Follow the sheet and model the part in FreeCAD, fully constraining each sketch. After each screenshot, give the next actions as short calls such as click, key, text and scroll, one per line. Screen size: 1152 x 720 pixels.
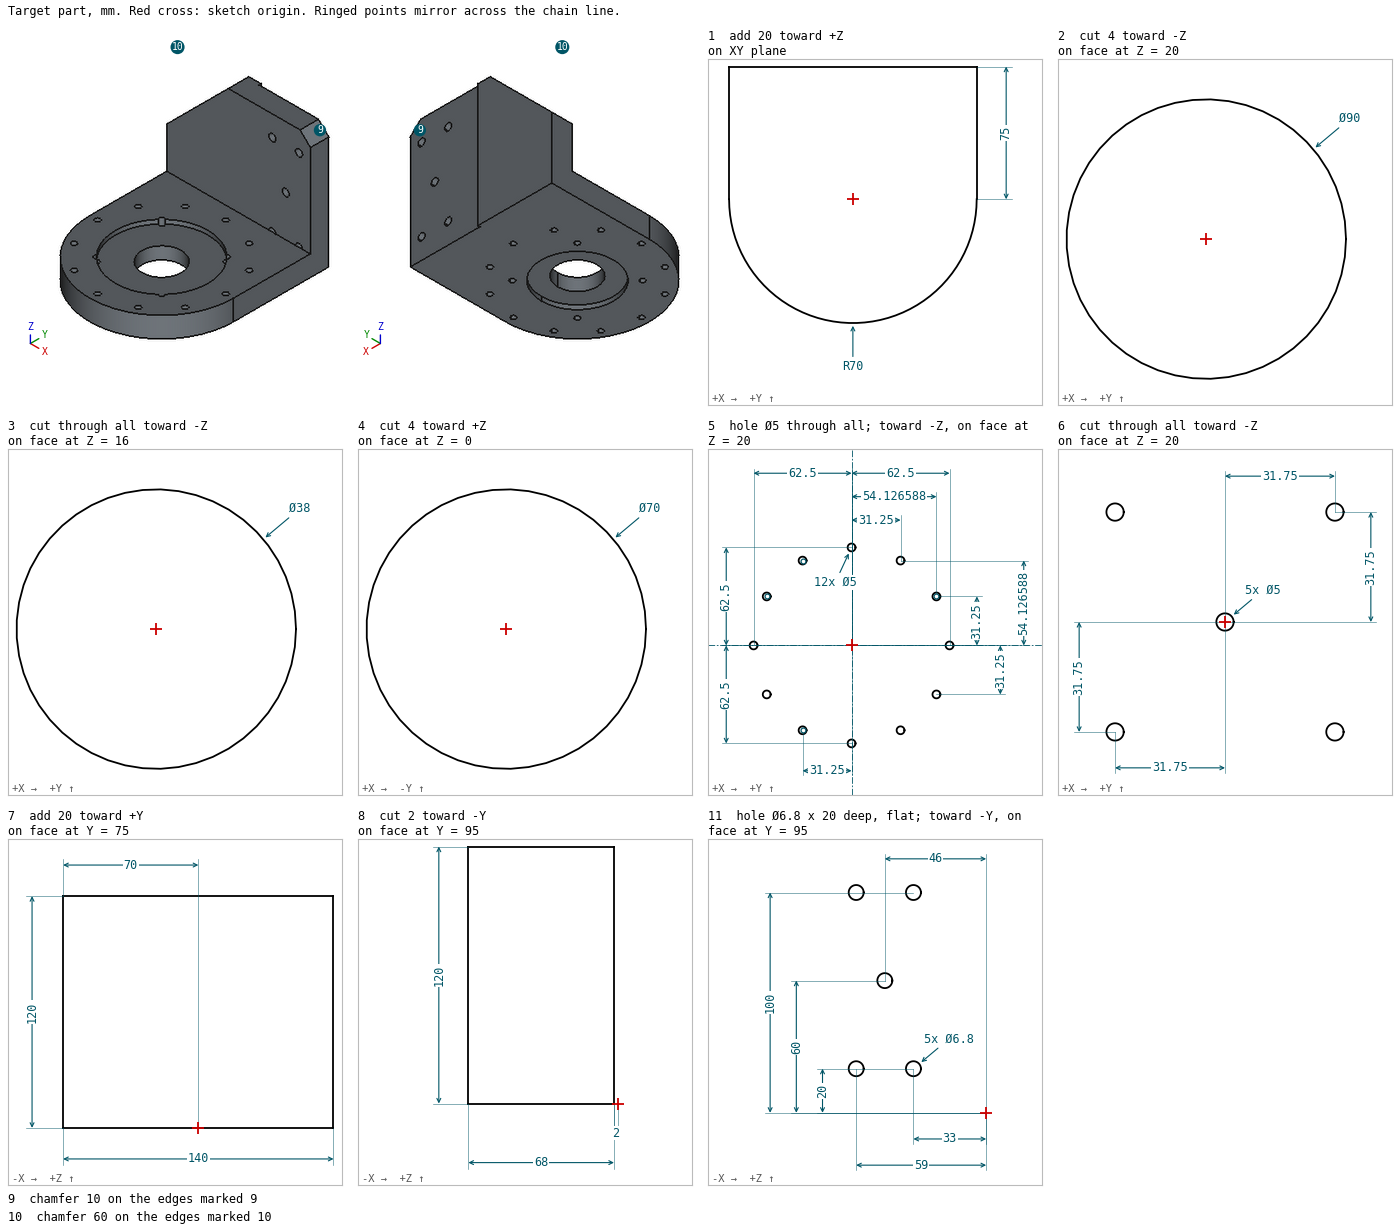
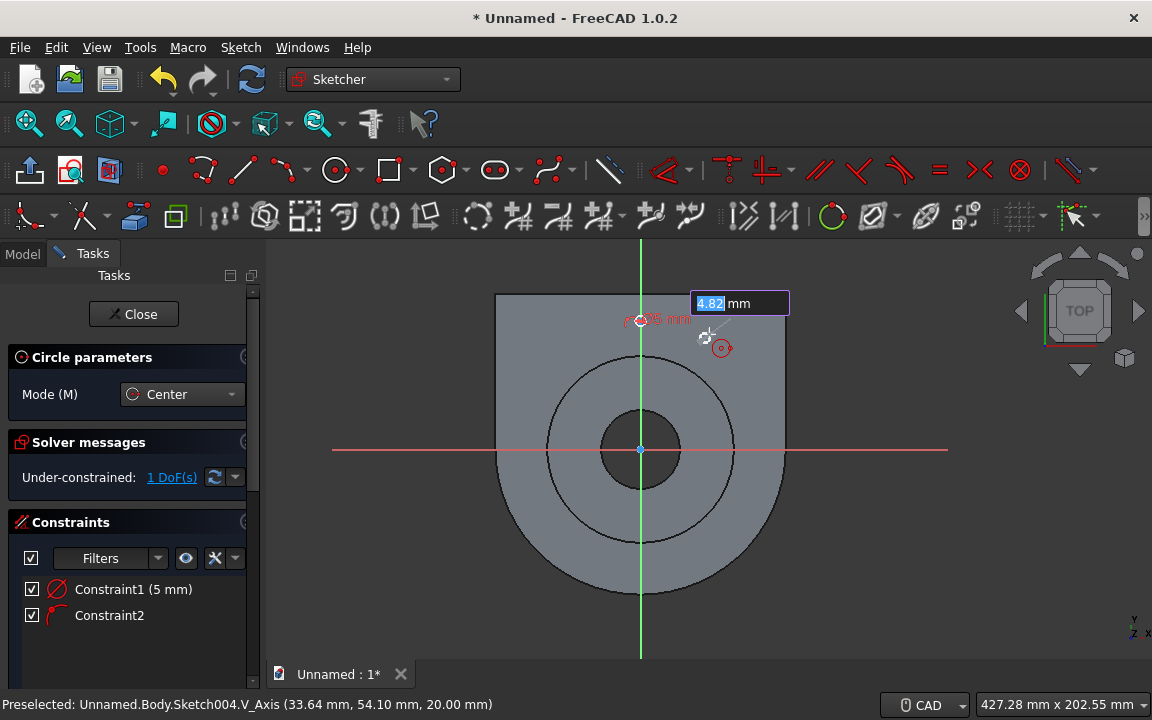
text(5)
key(Return)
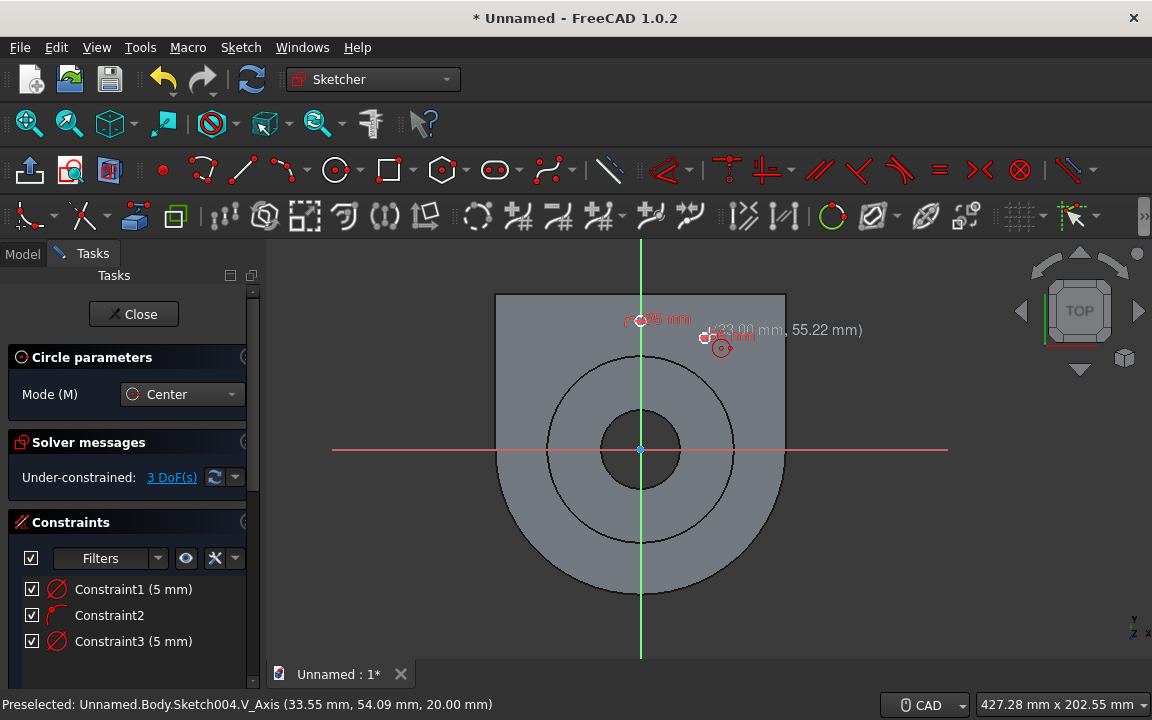
scroll(753, 385, up, 8)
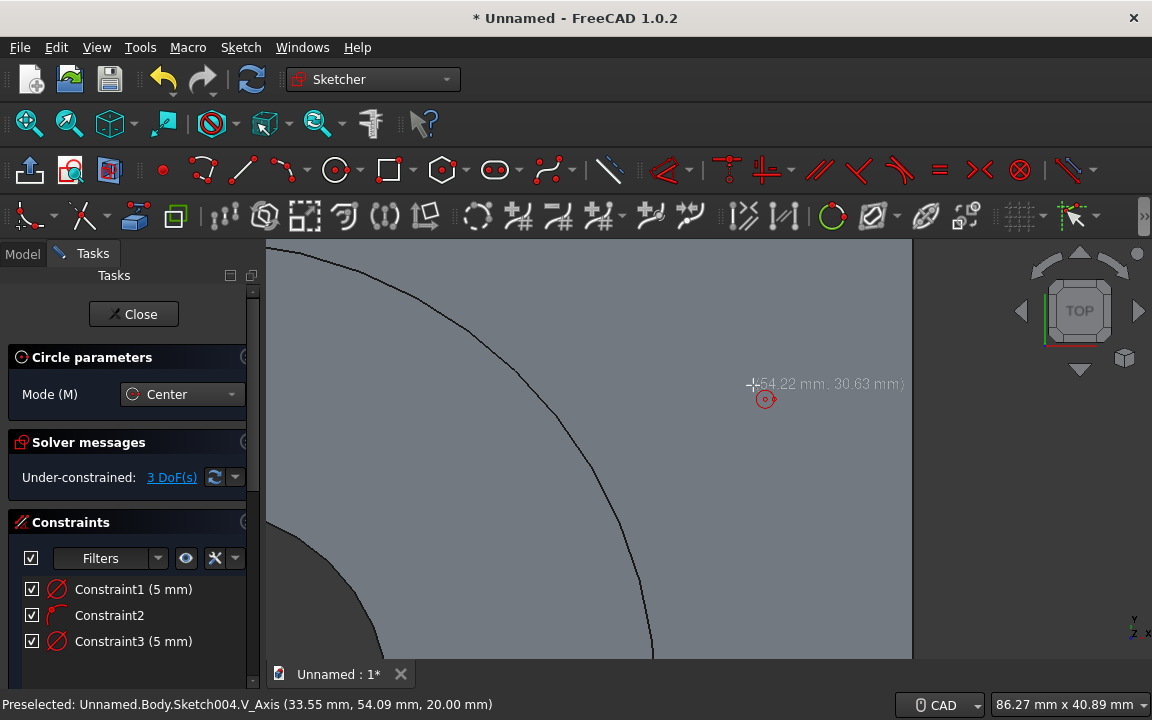
scroll(753, 385, down, 8)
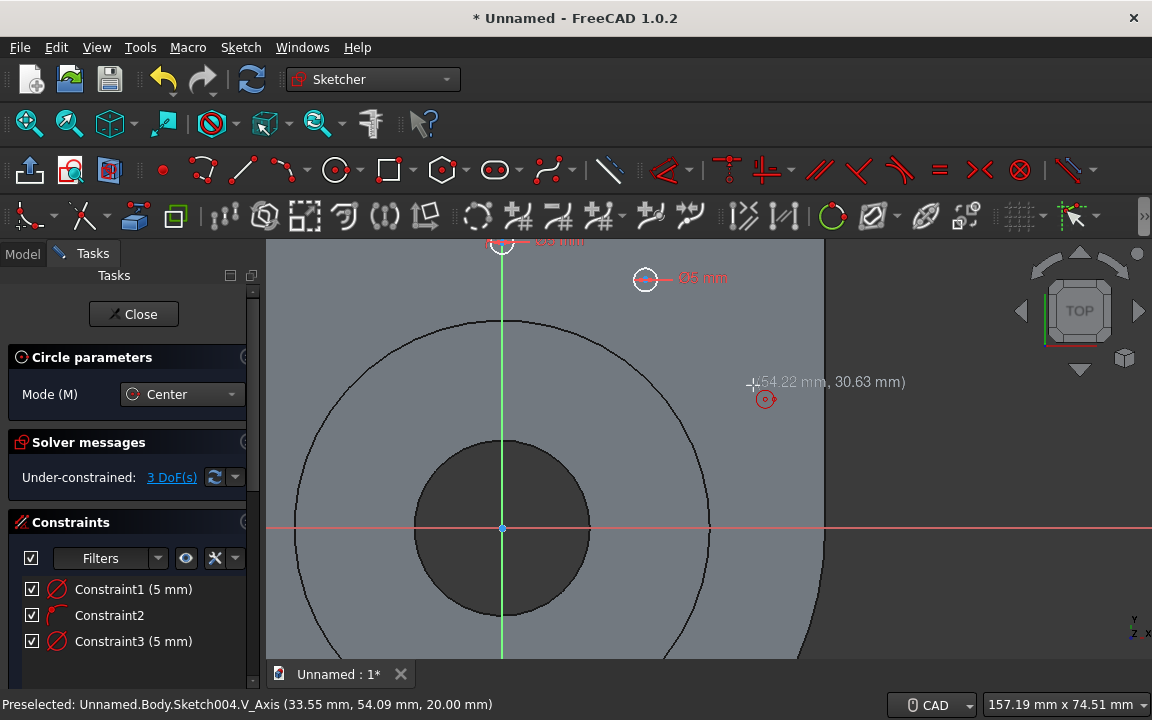
click(753, 385)
move(756, 381)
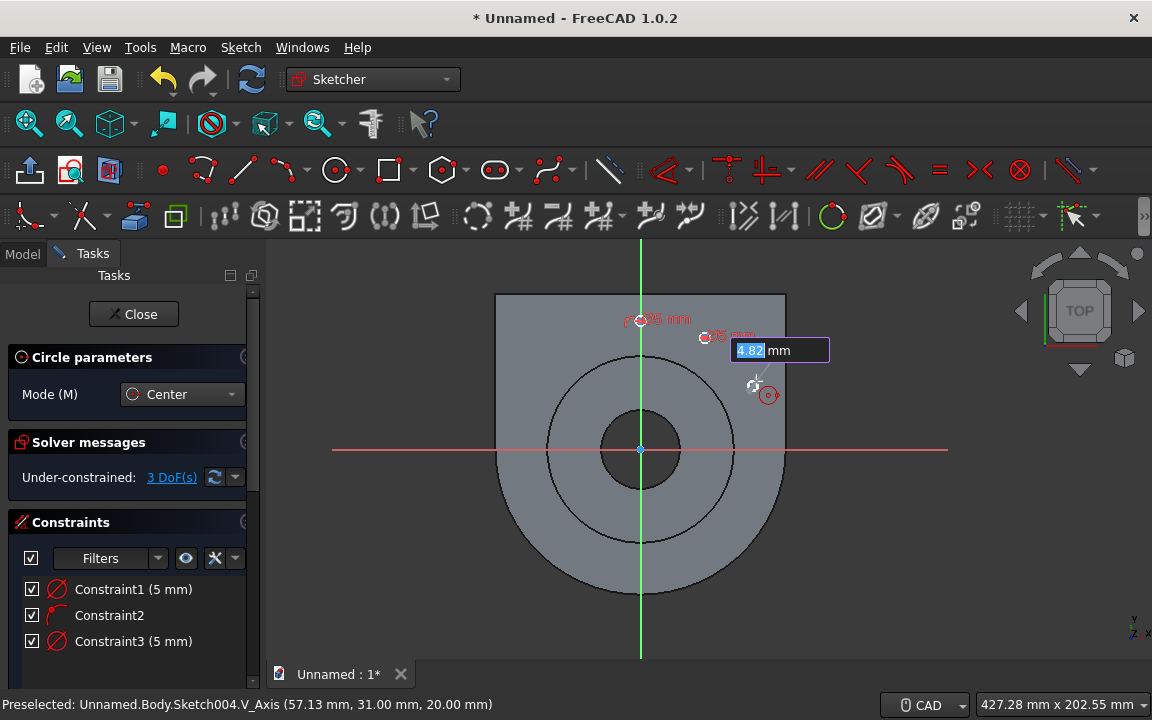
text(5)
key(Return)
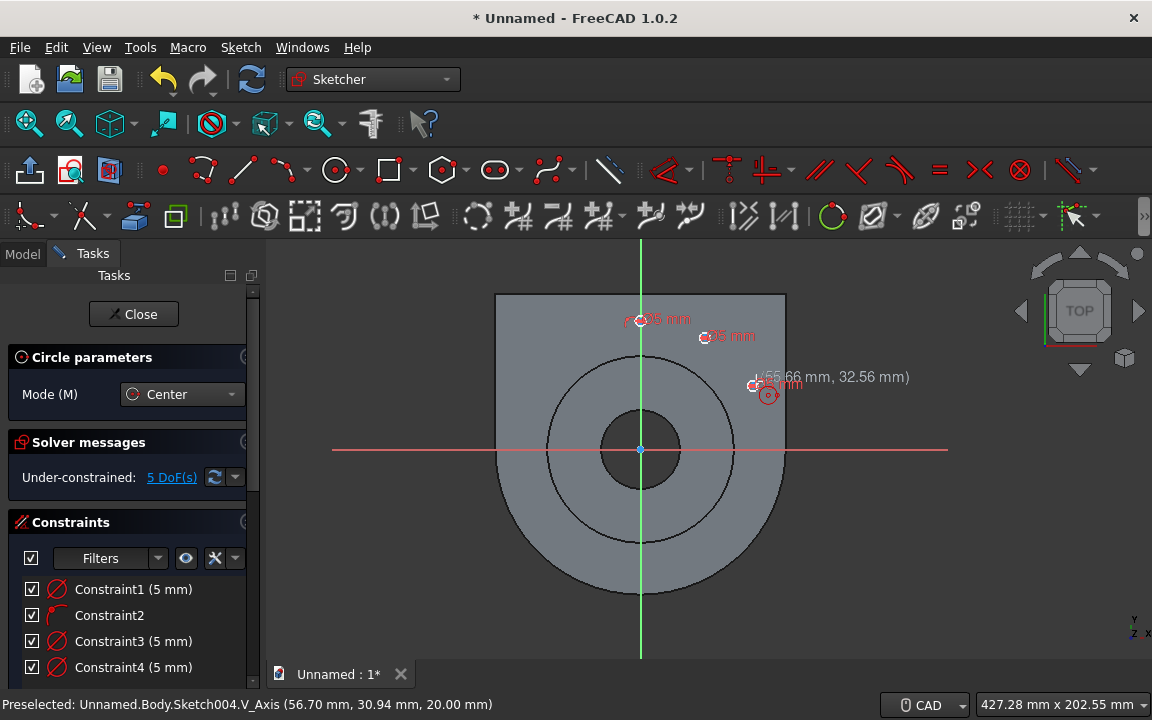
scroll(770, 450, up, 8)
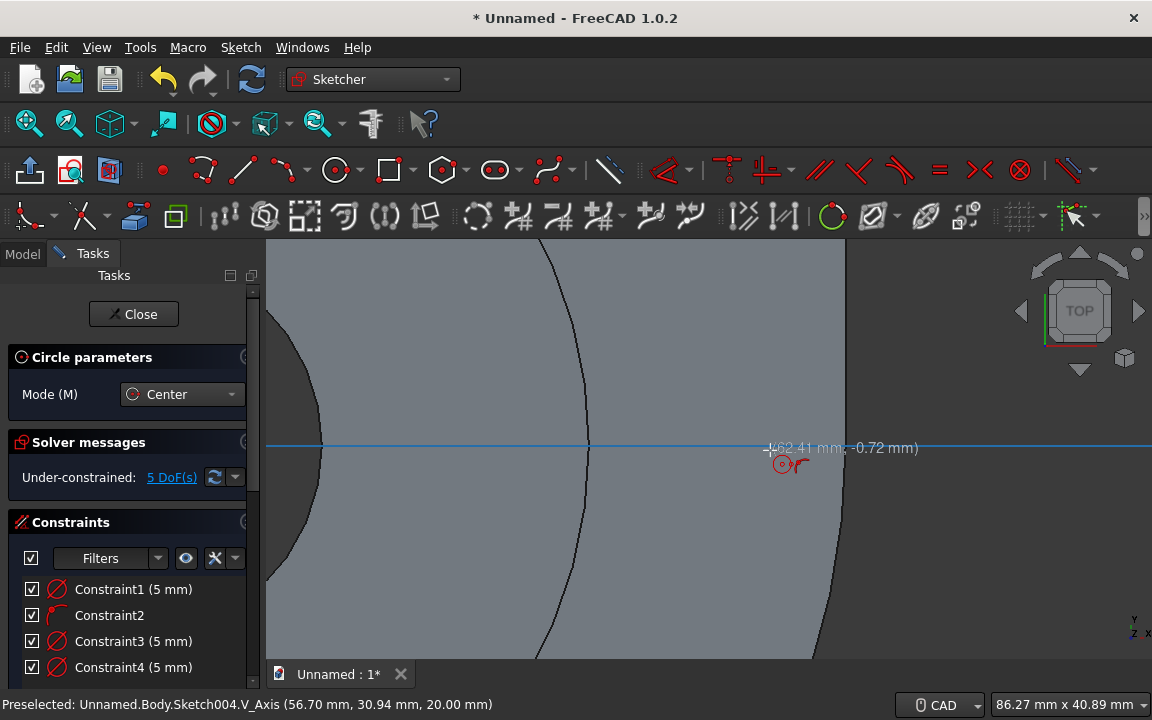
scroll(770, 450, down, 8)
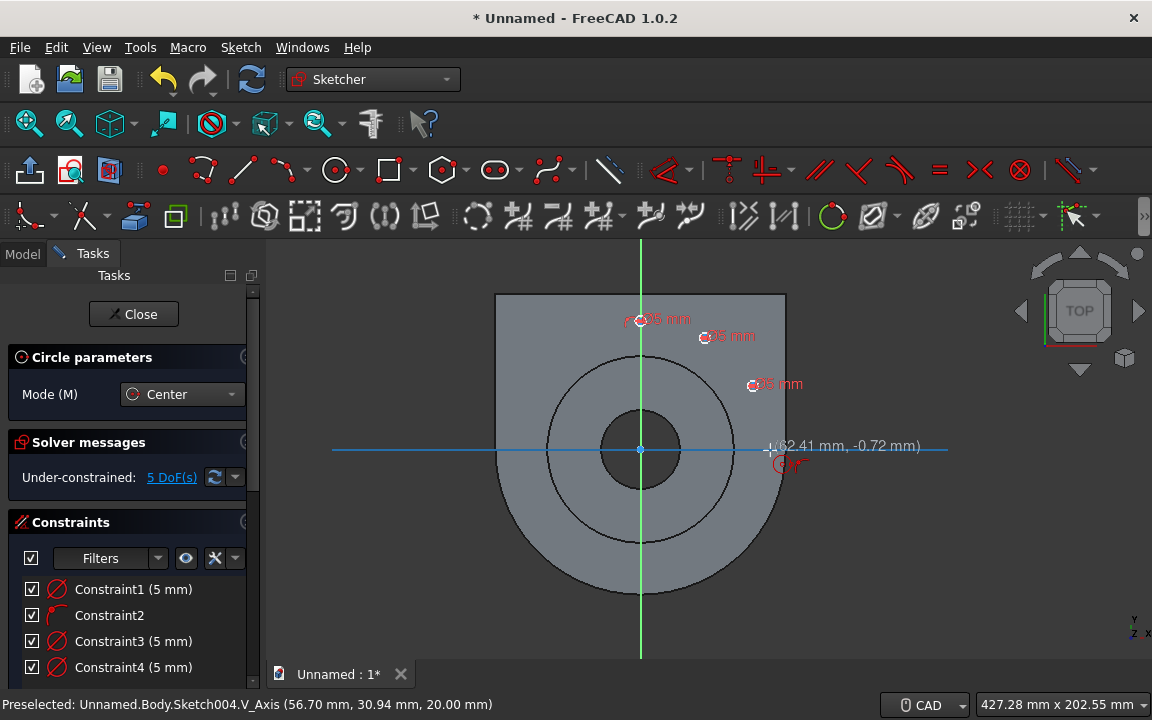
click(770, 450)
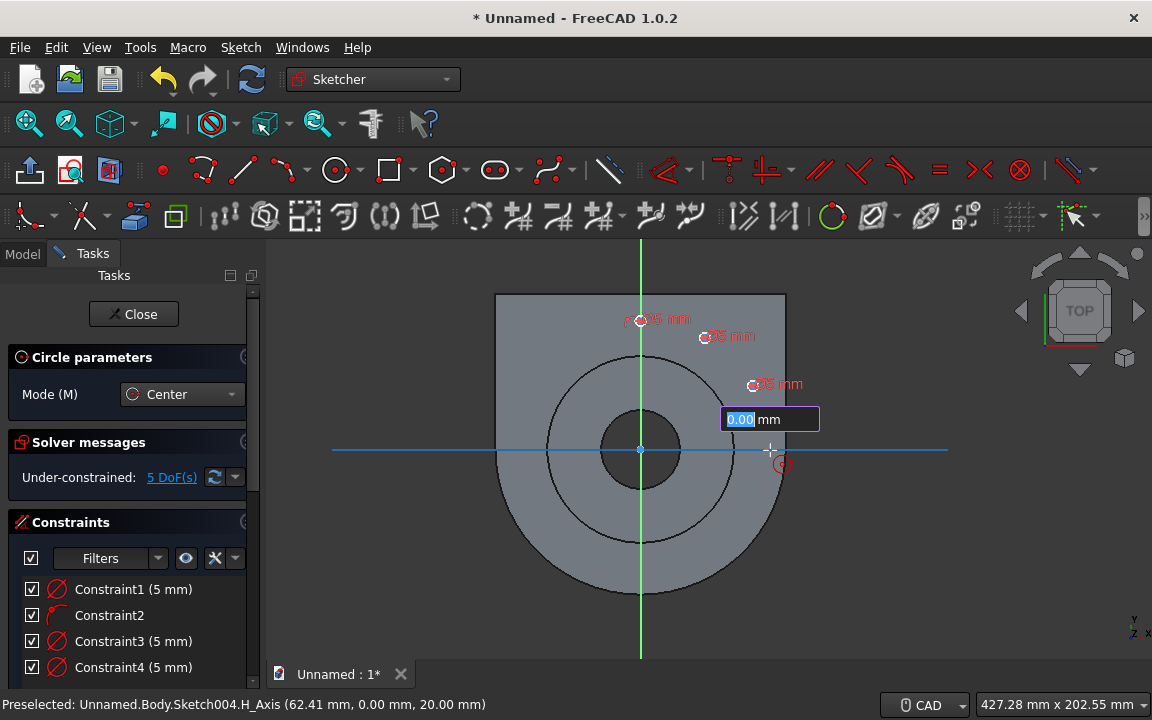
scroll(768, 454, up, 6)
move(768, 454)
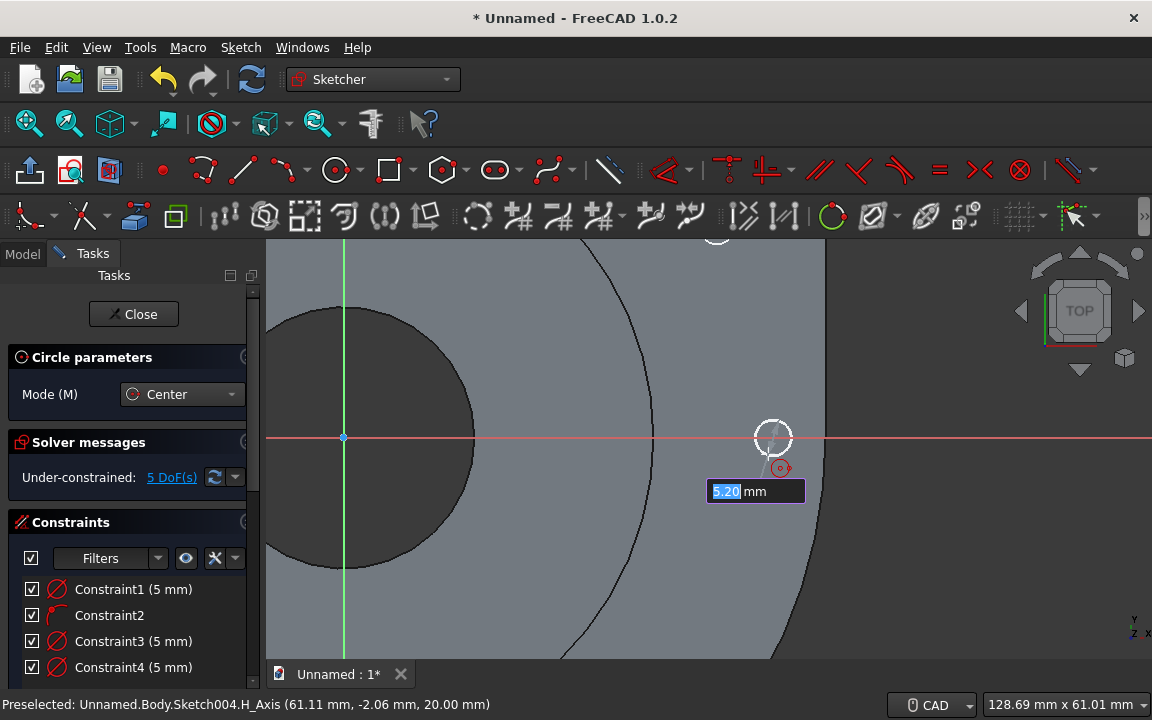
text(5)
key(Return)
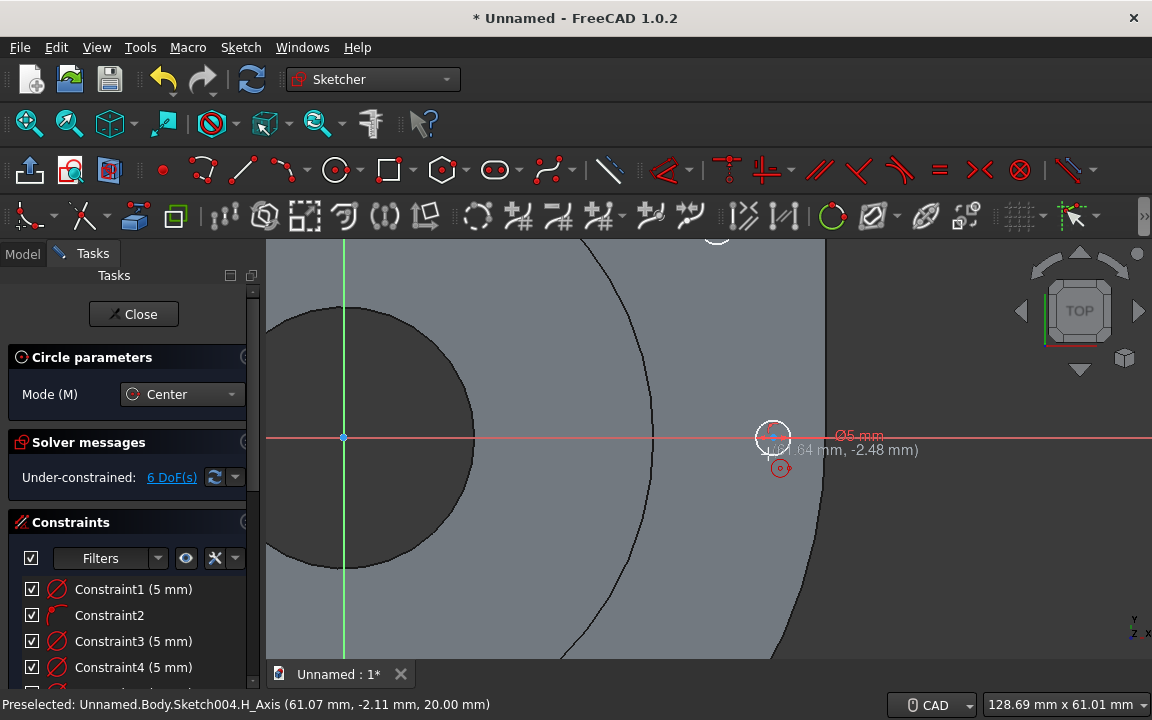
scroll(768, 454, down, 6)